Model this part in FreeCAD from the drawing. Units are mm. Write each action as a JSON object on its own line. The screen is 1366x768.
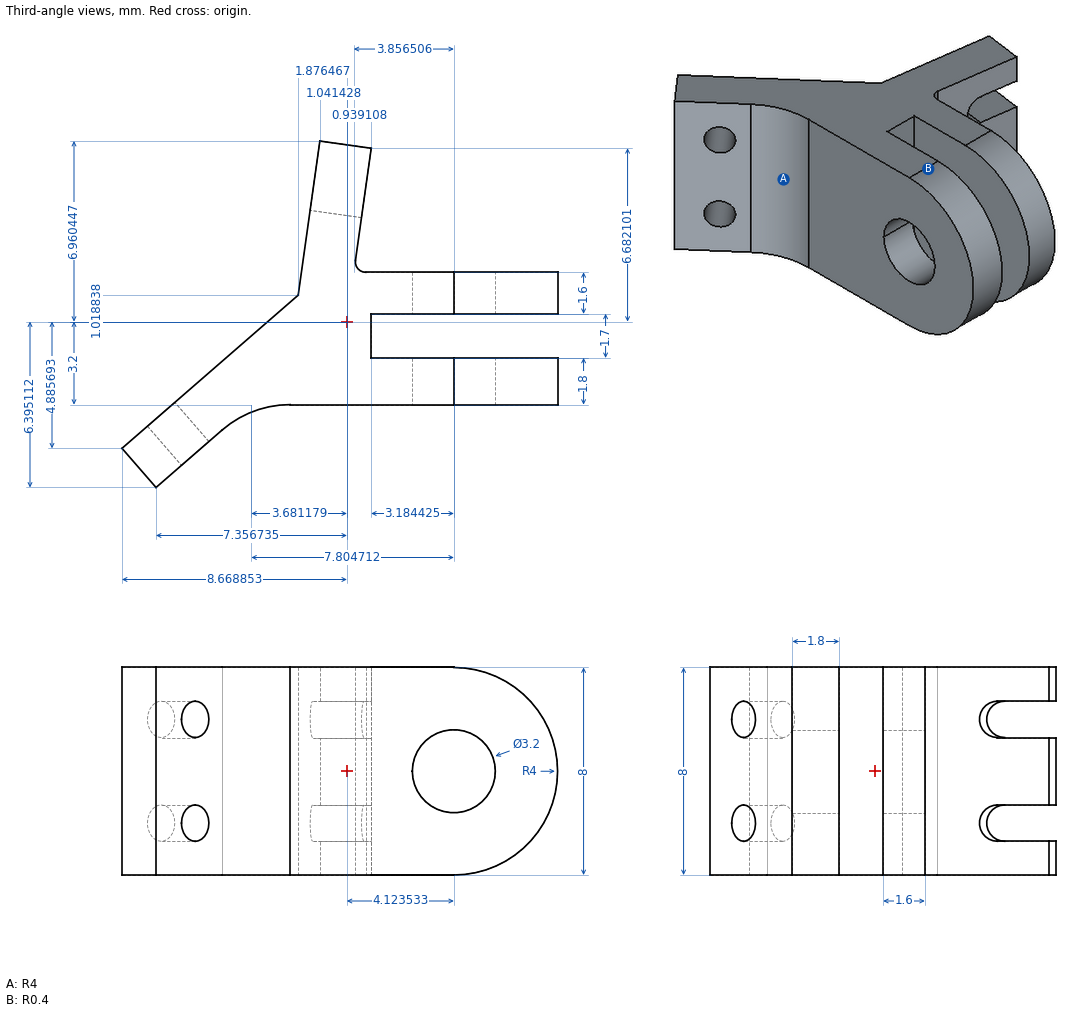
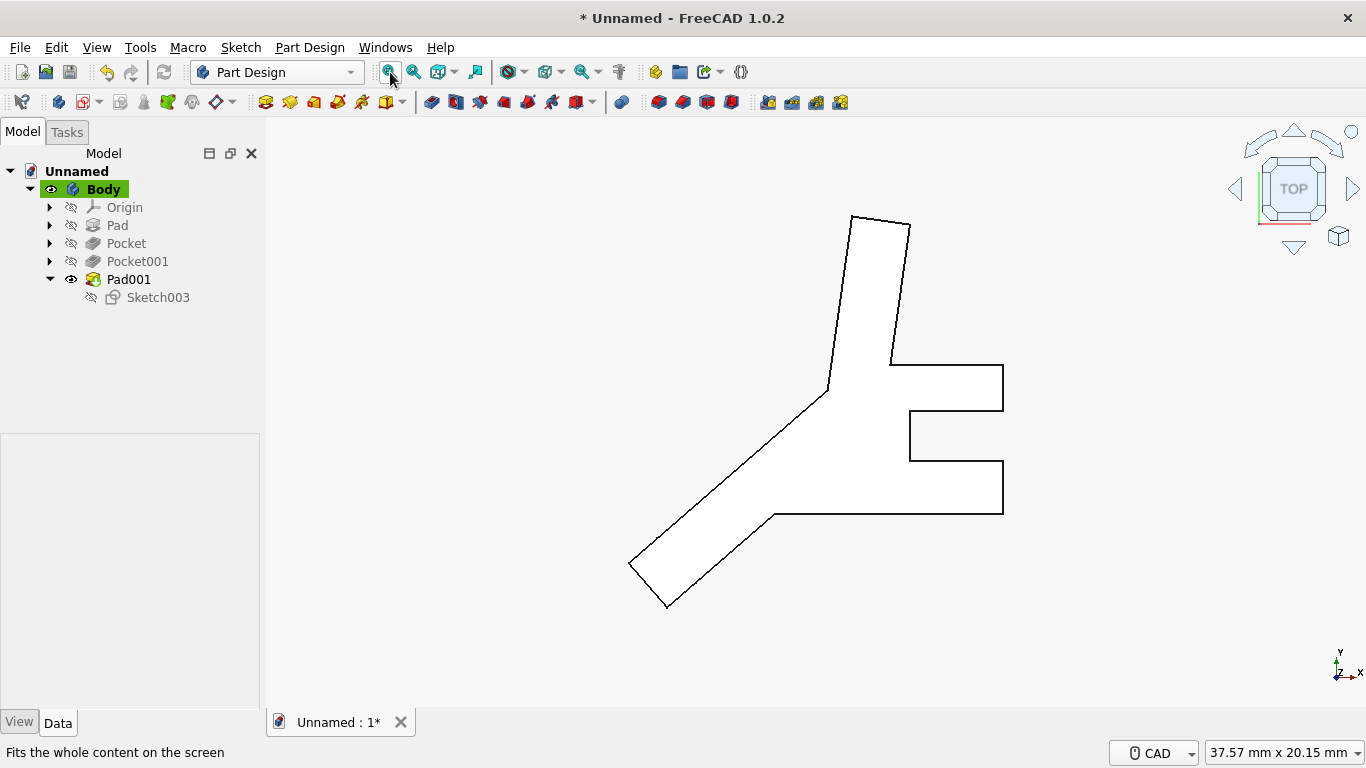
{"action": "key", "text": "1"}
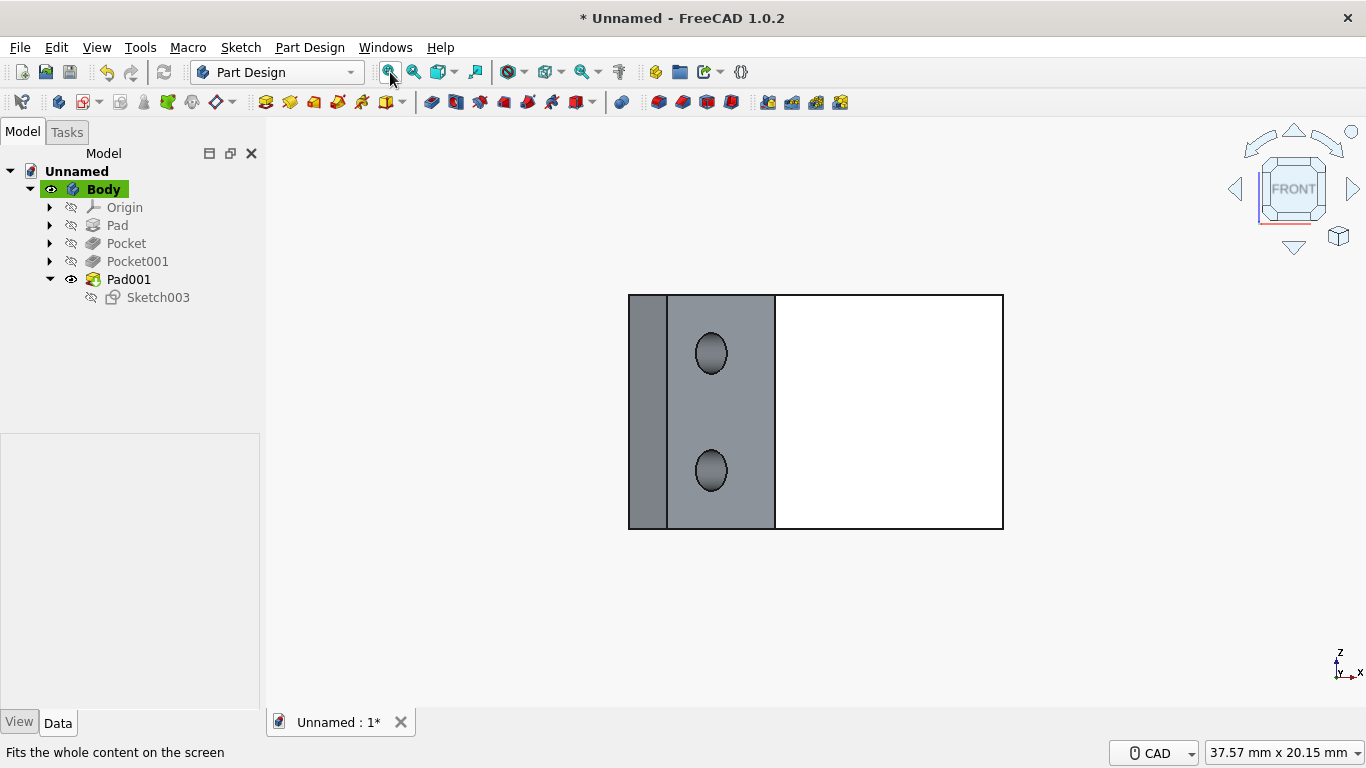
{"action": "left_click", "coordinate": [390, 72]}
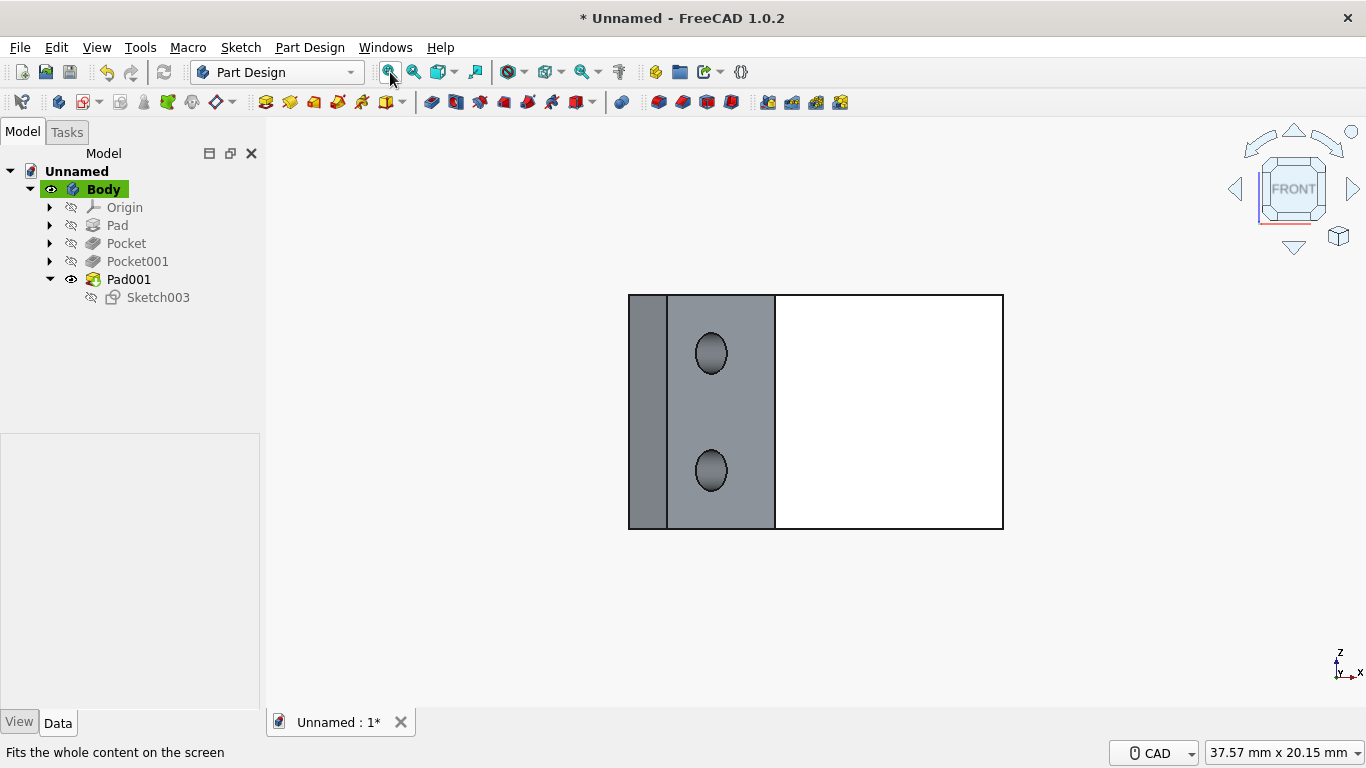
{"action": "key", "text": "3"}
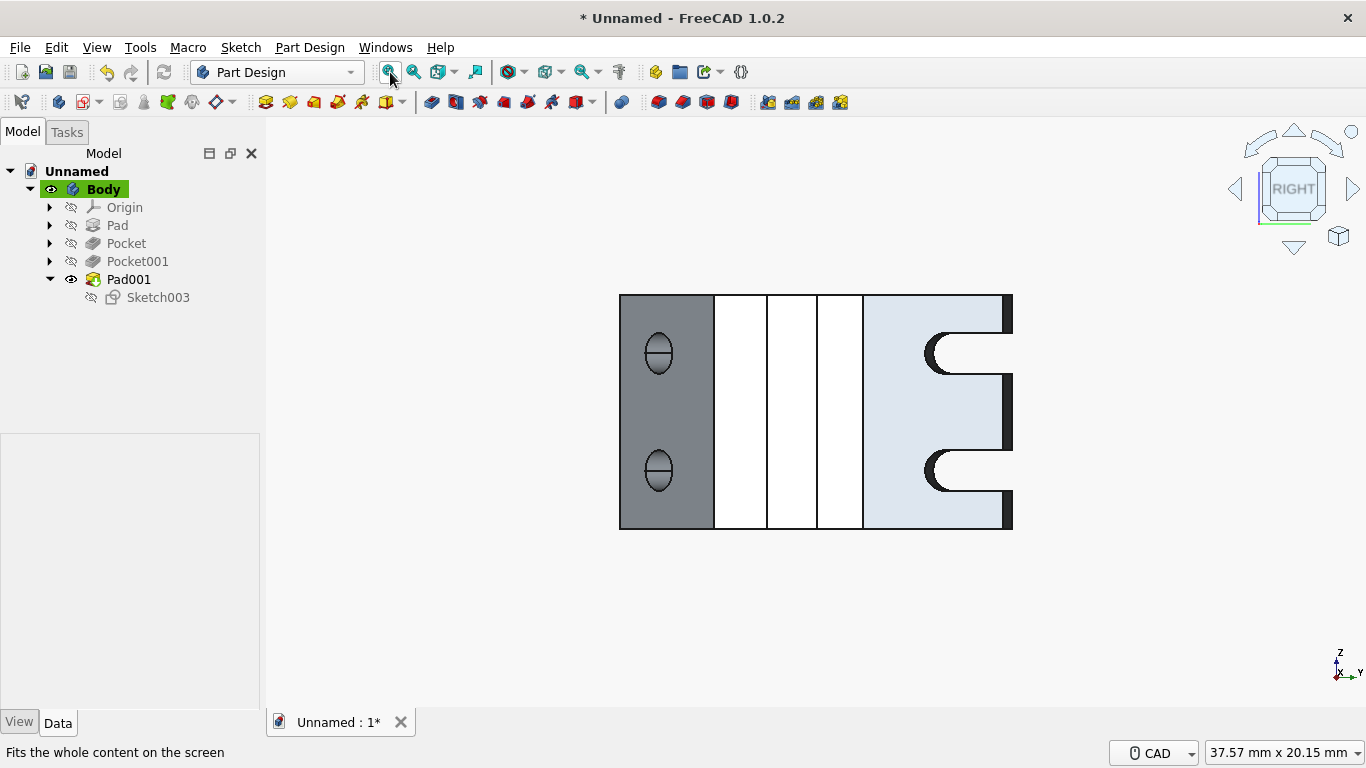
{"action": "left_click", "coordinate": [390, 72]}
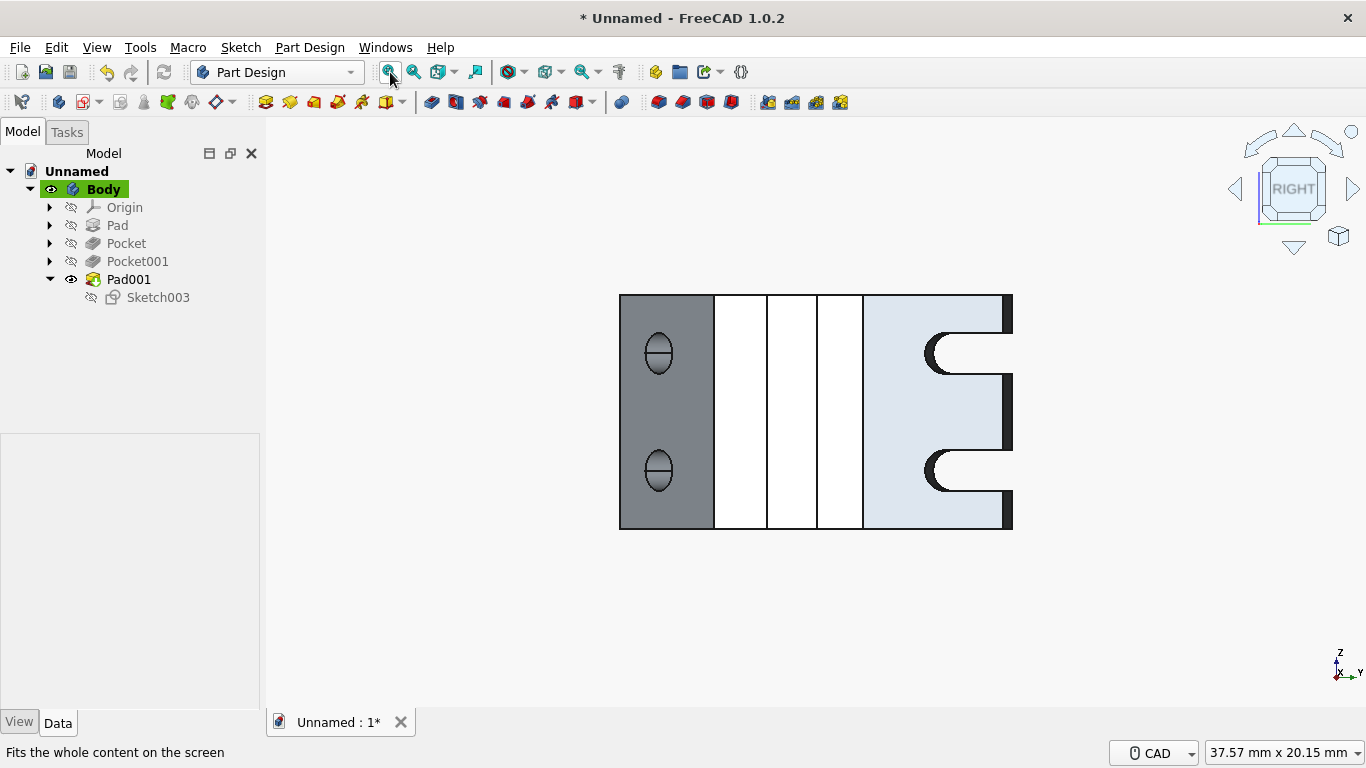
{"action": "key", "text": "5"}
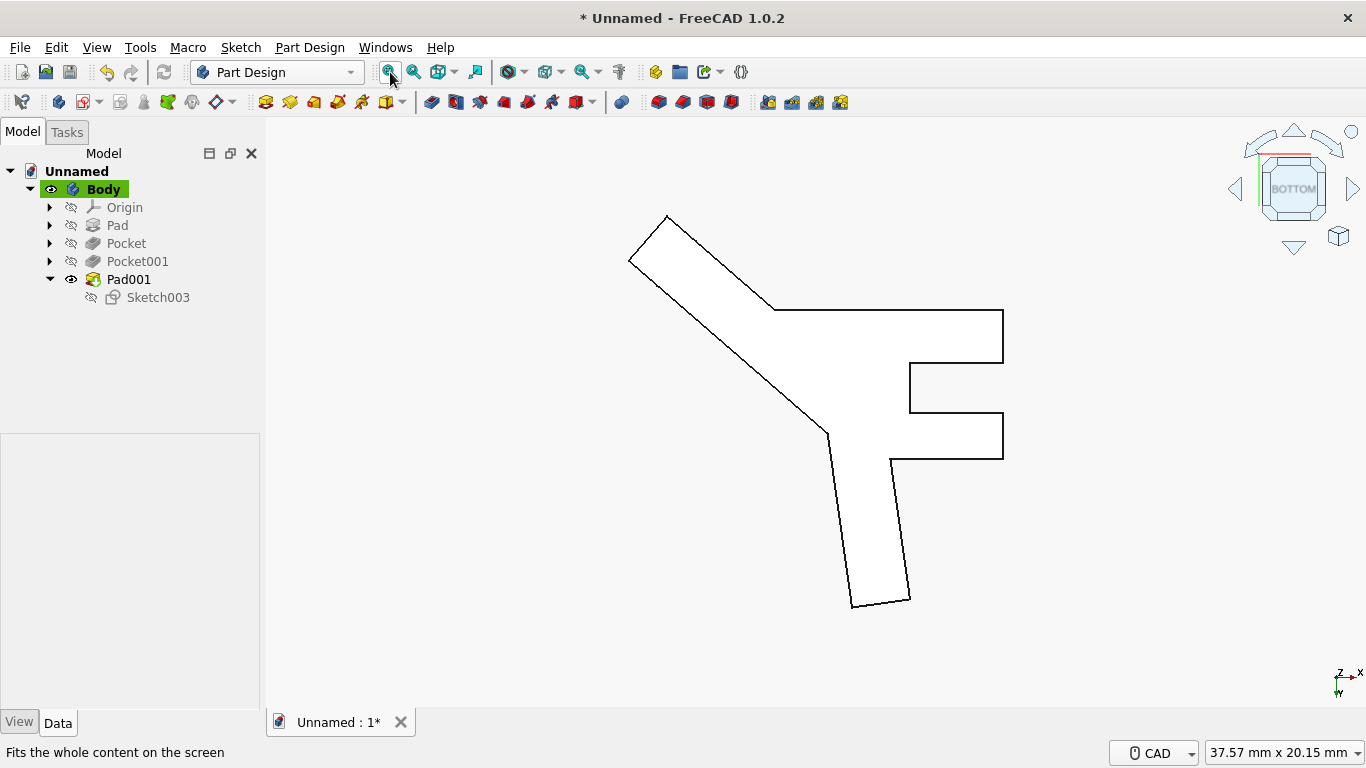
{"action": "key", "text": "4"}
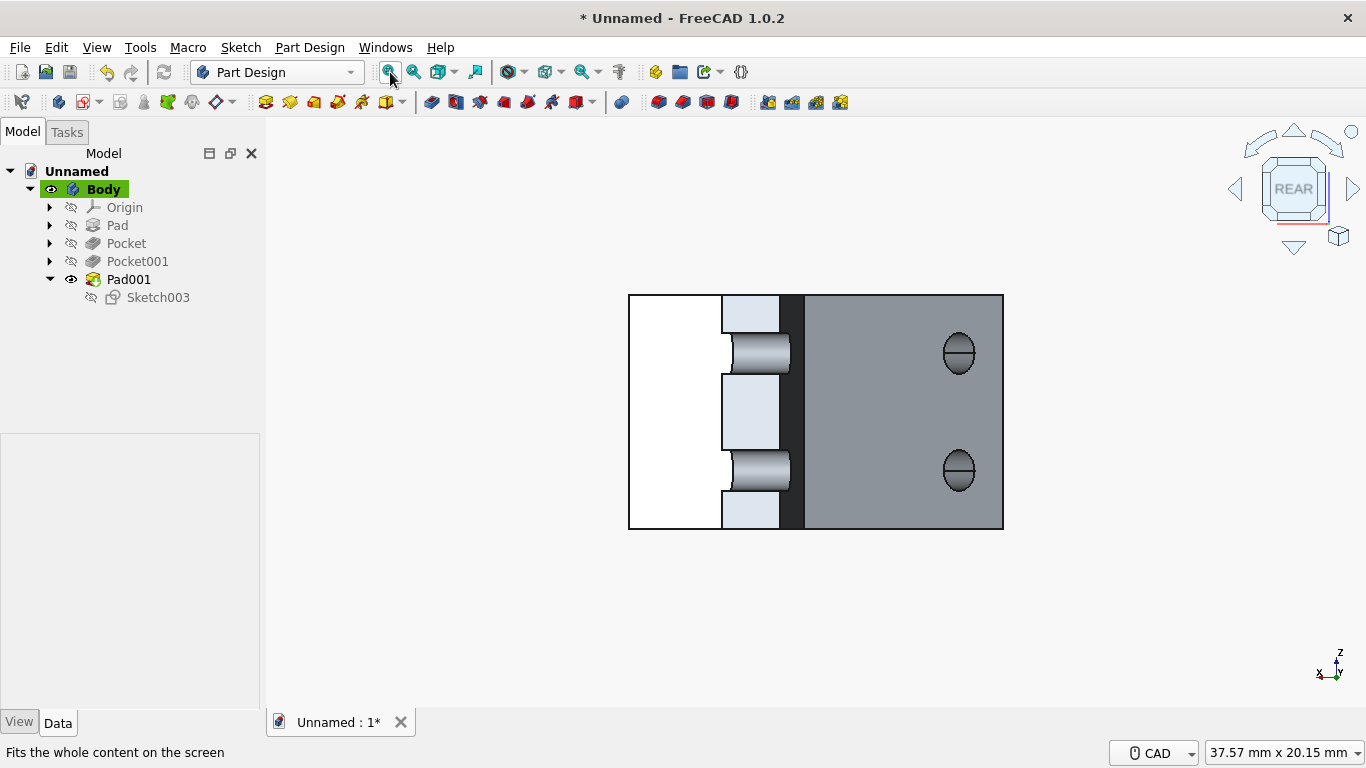
{"action": "left_click", "coordinate": [390, 72]}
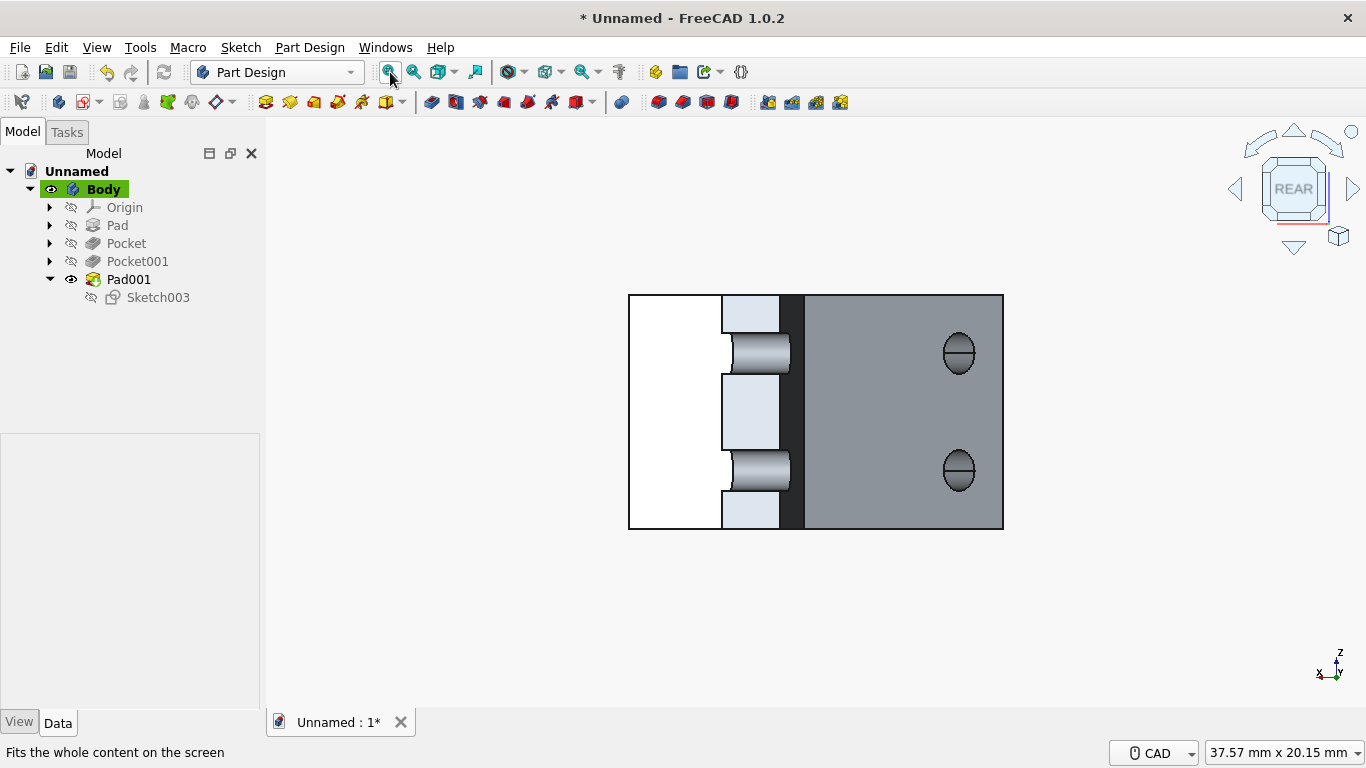
{"action": "key", "text": "6"}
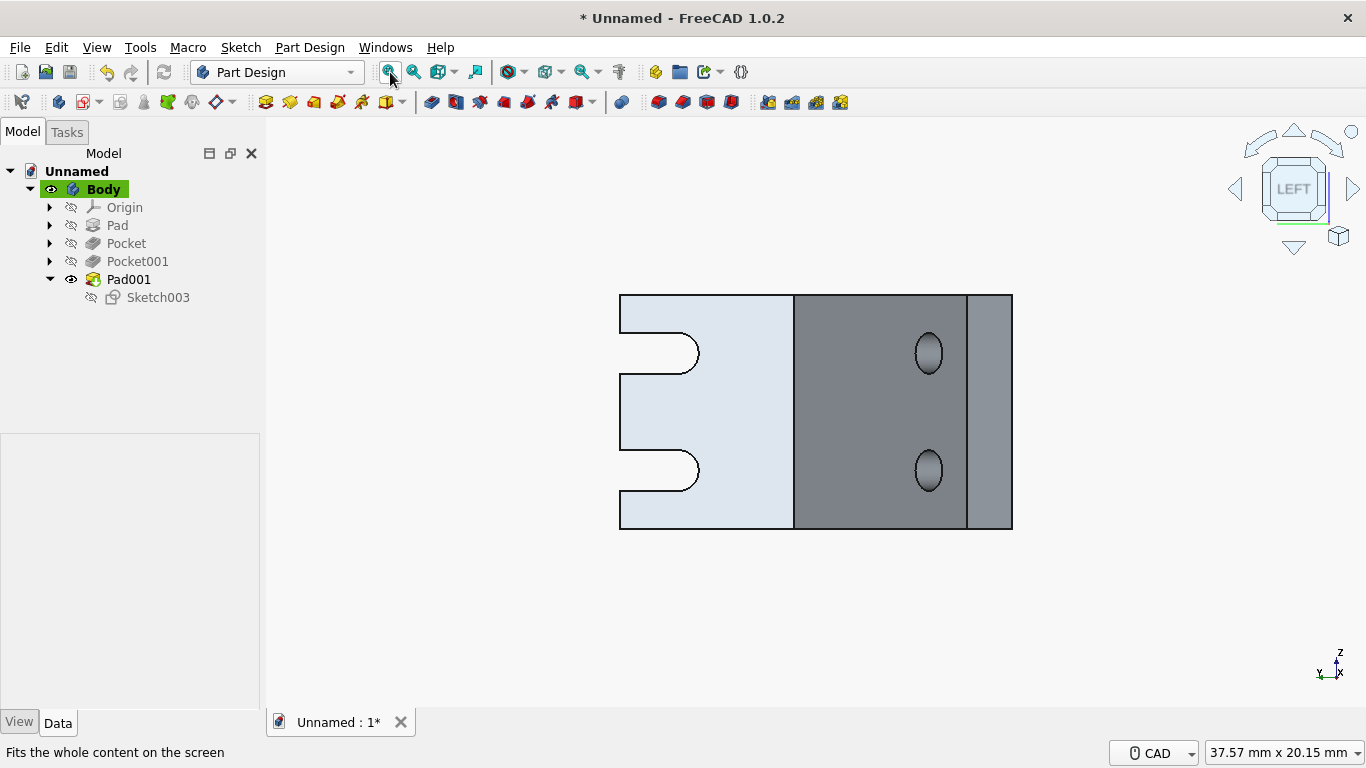
{"action": "left_click", "coordinate": [390, 72]}